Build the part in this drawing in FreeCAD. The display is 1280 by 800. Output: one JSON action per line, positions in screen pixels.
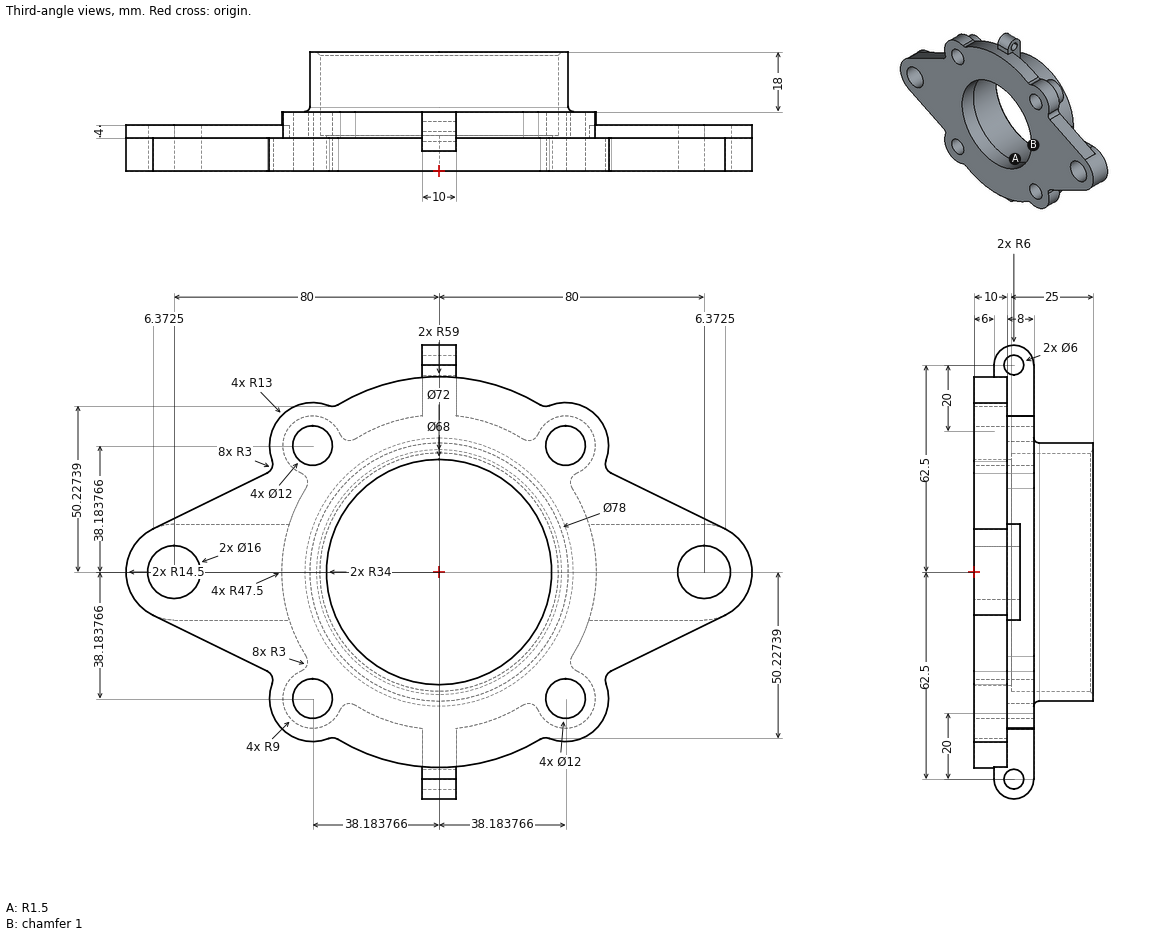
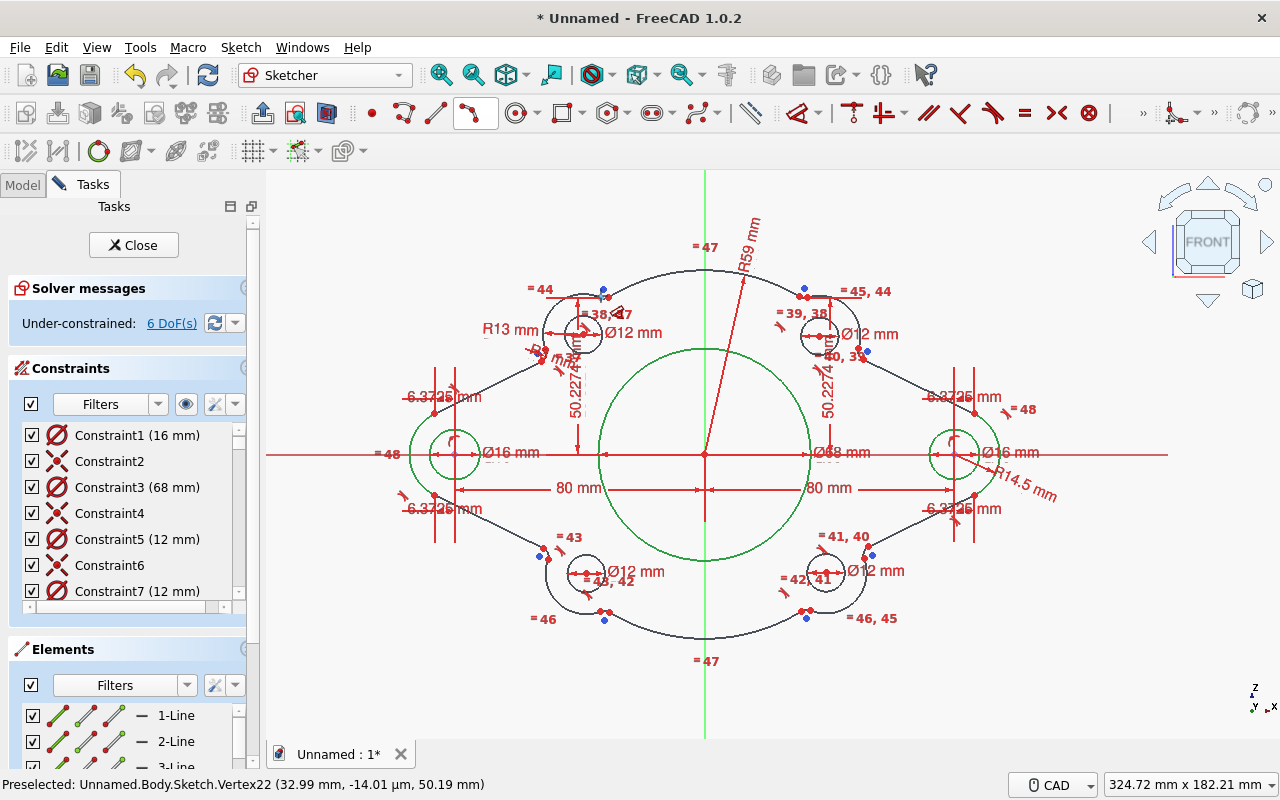
{"action": "scroll", "coordinate": [810, 610], "scroll_direction": "up", "scroll_amount": 2}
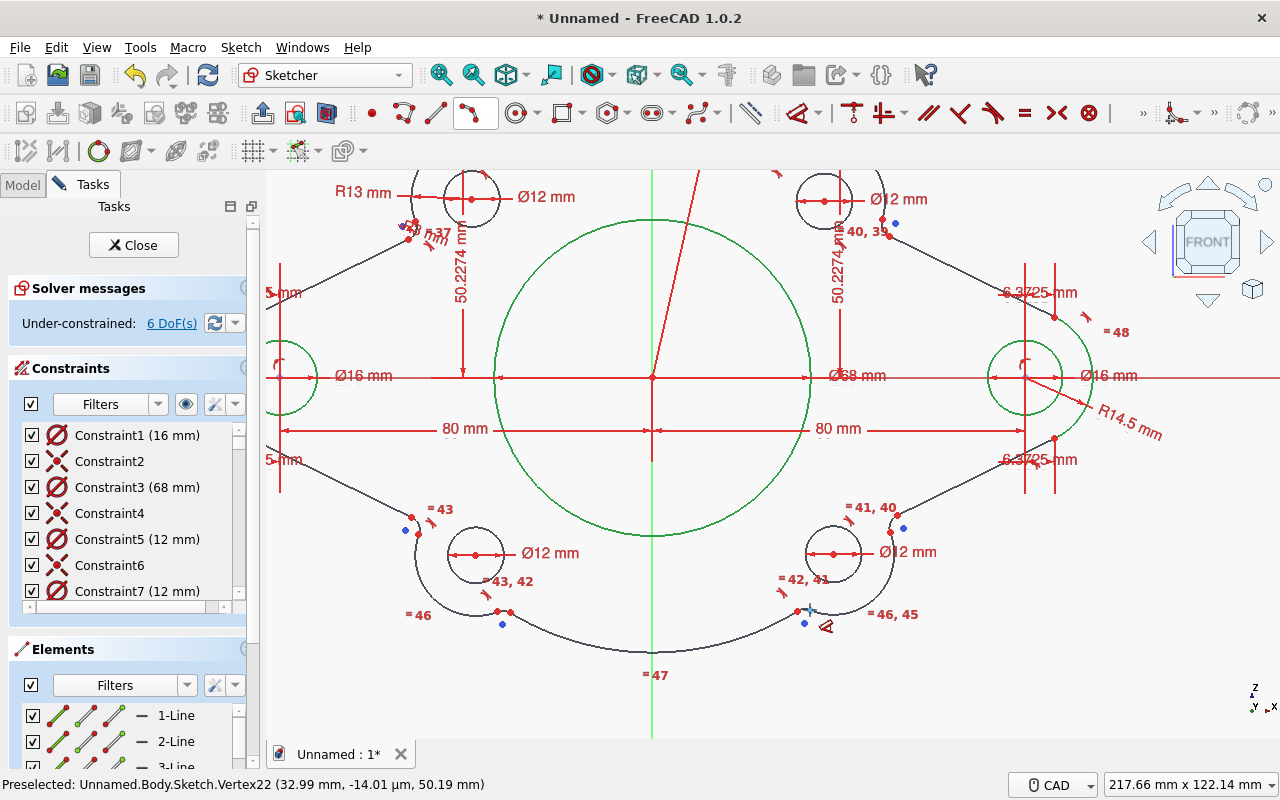
{"action": "left_click", "coordinate": [810, 610]}
{"action": "left_click", "coordinate": [844, 494]}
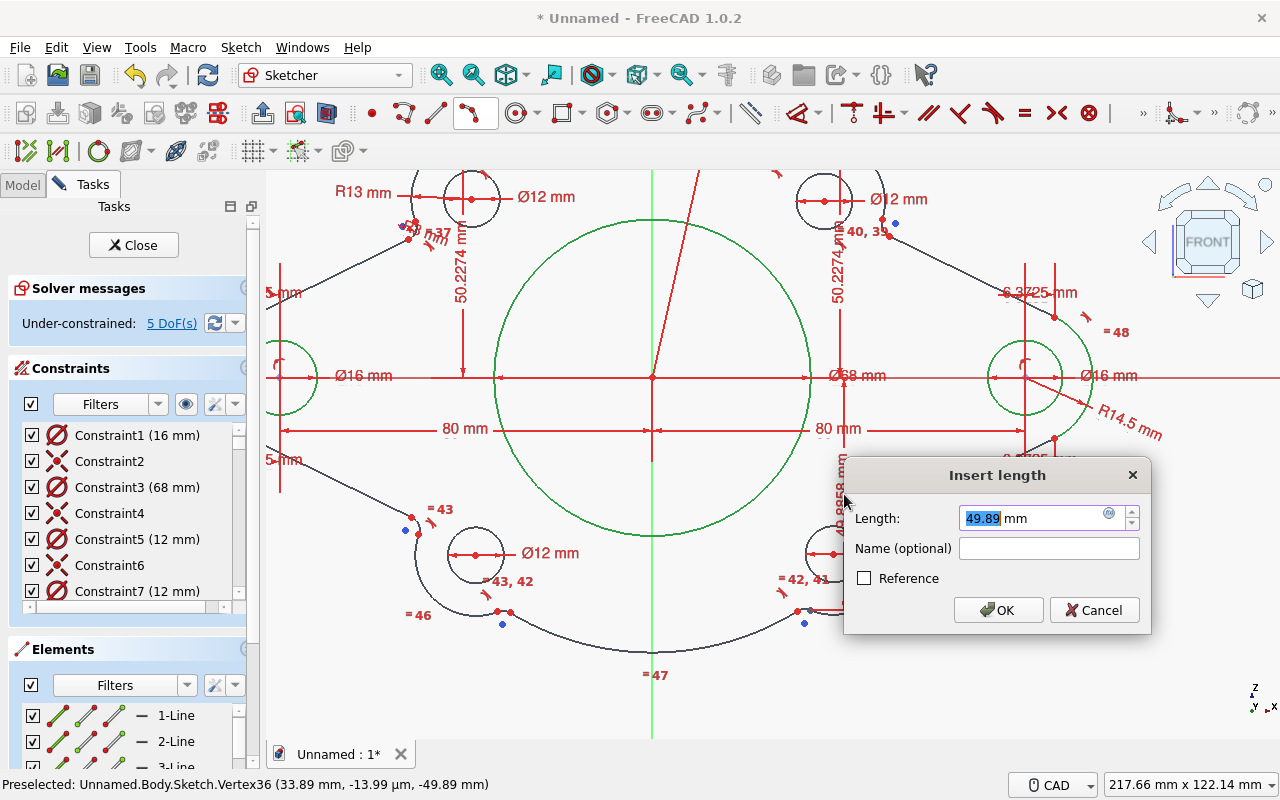
{"action": "type", "text": "50.22739"}
{"action": "key", "text": "Return"}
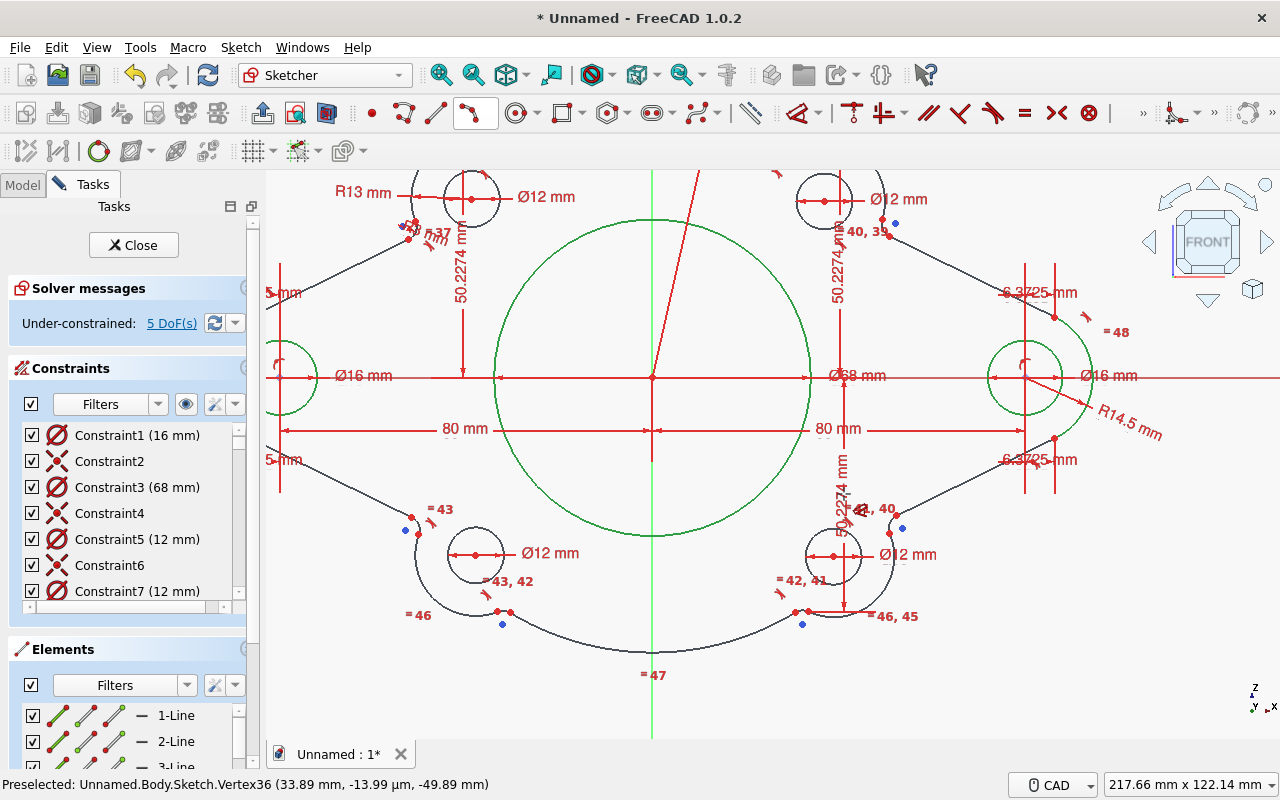
{"action": "left_click", "coordinate": [498, 612]}
{"action": "left_click", "coordinate": [464, 495]}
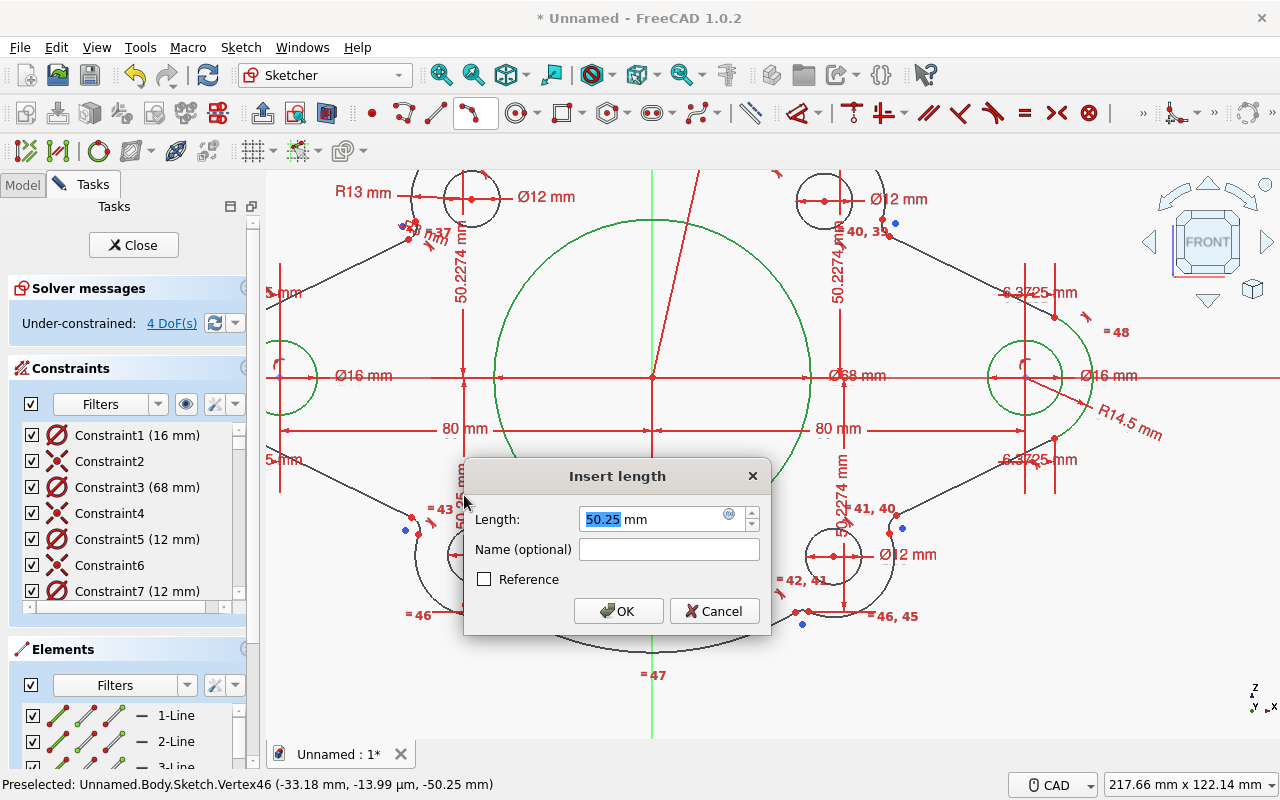
{"action": "type", "text": "50.22739"}
{"action": "key", "text": "Return"}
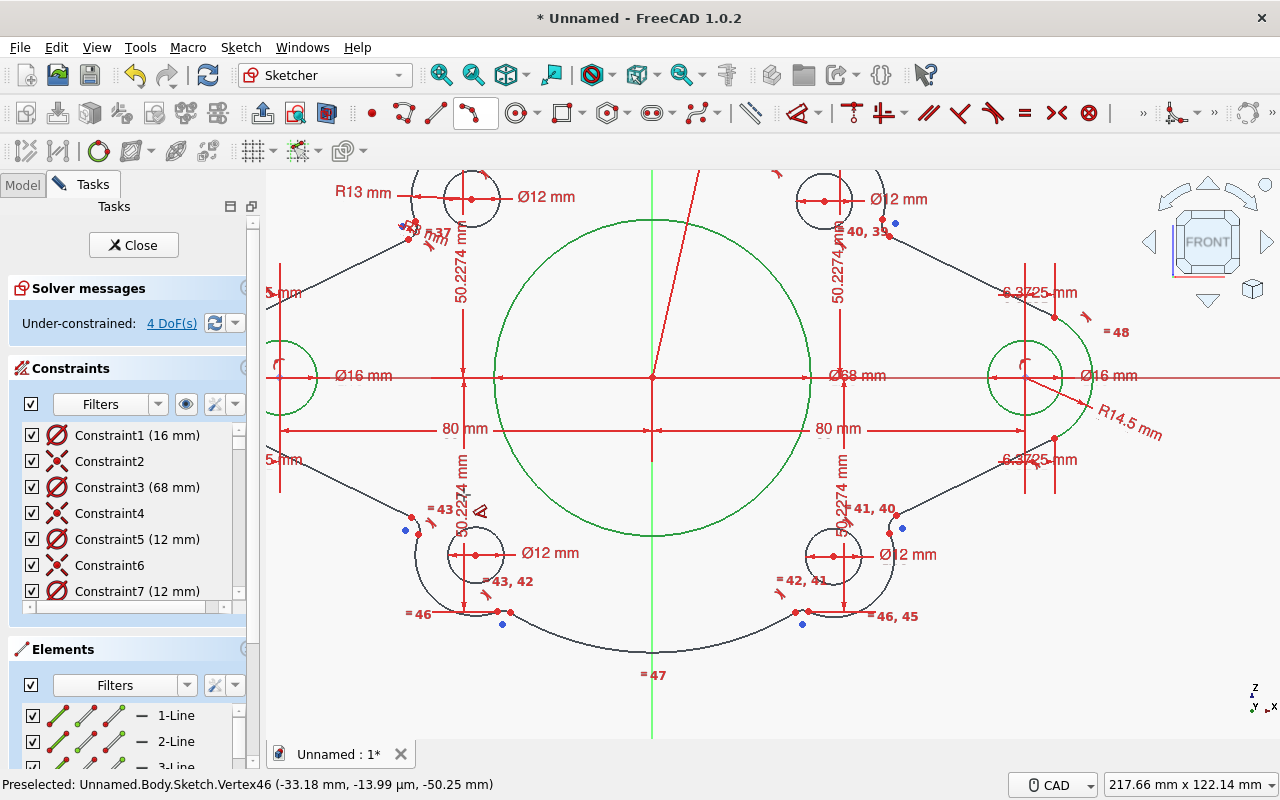
{"action": "left_click", "coordinate": [834, 557]}
{"action": "left_click", "coordinate": [743, 591]}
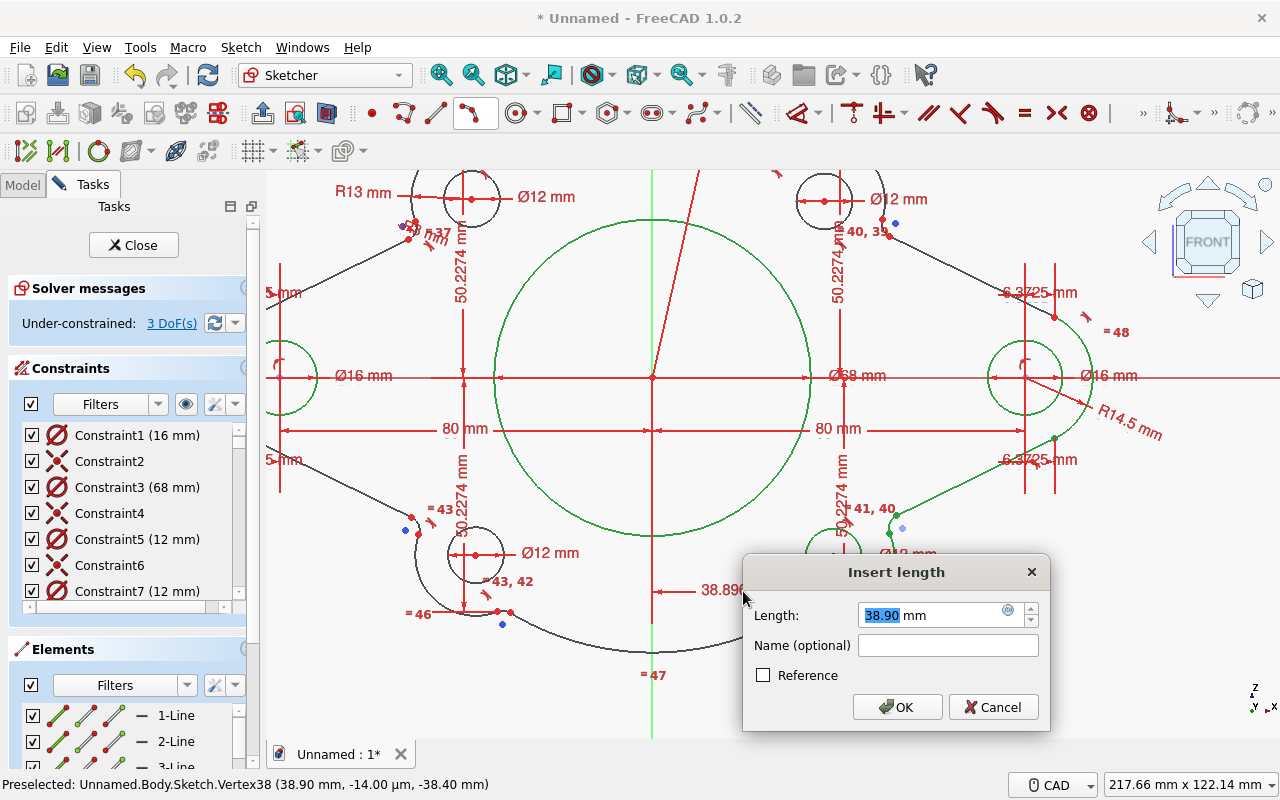
{"action": "type", "text": "38.183766"}
{"action": "key", "text": "Return"}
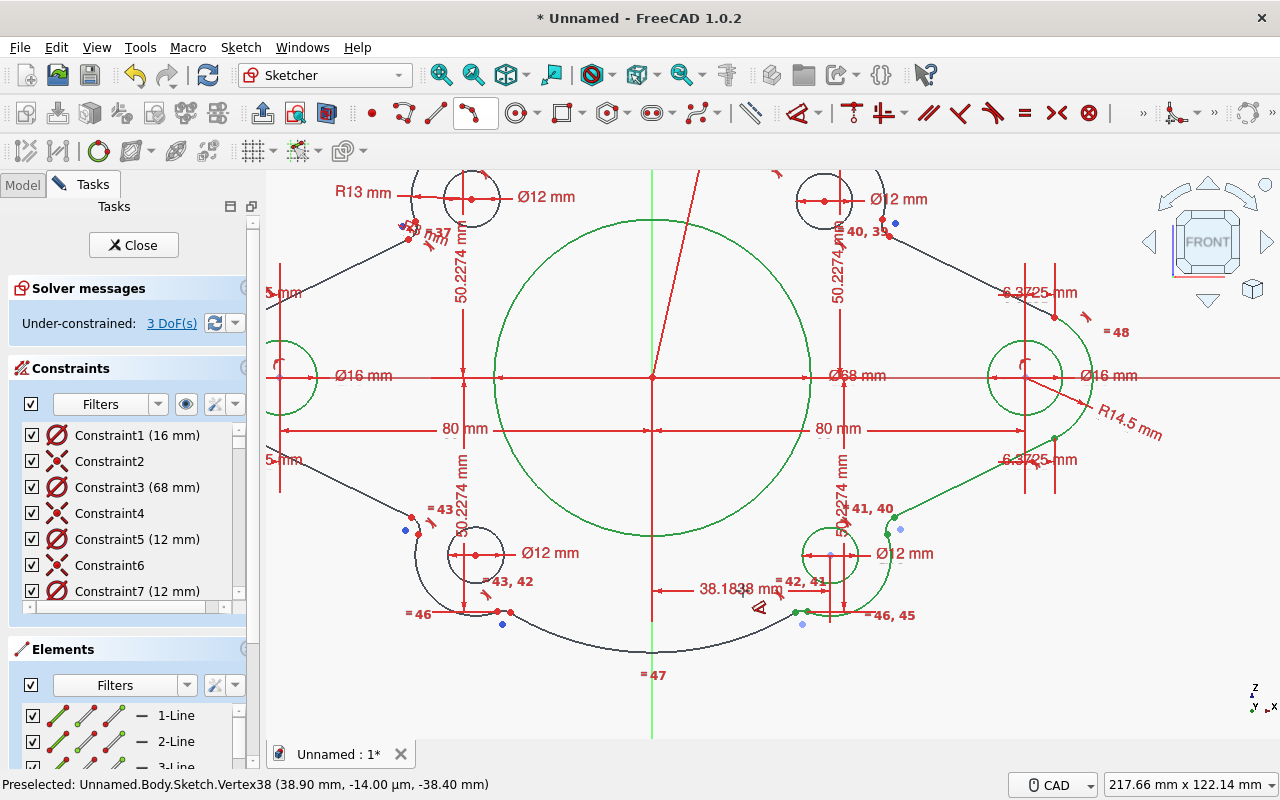
{"action": "left_click", "coordinate": [476, 555]}
{"action": "left_click", "coordinate": [564, 589]}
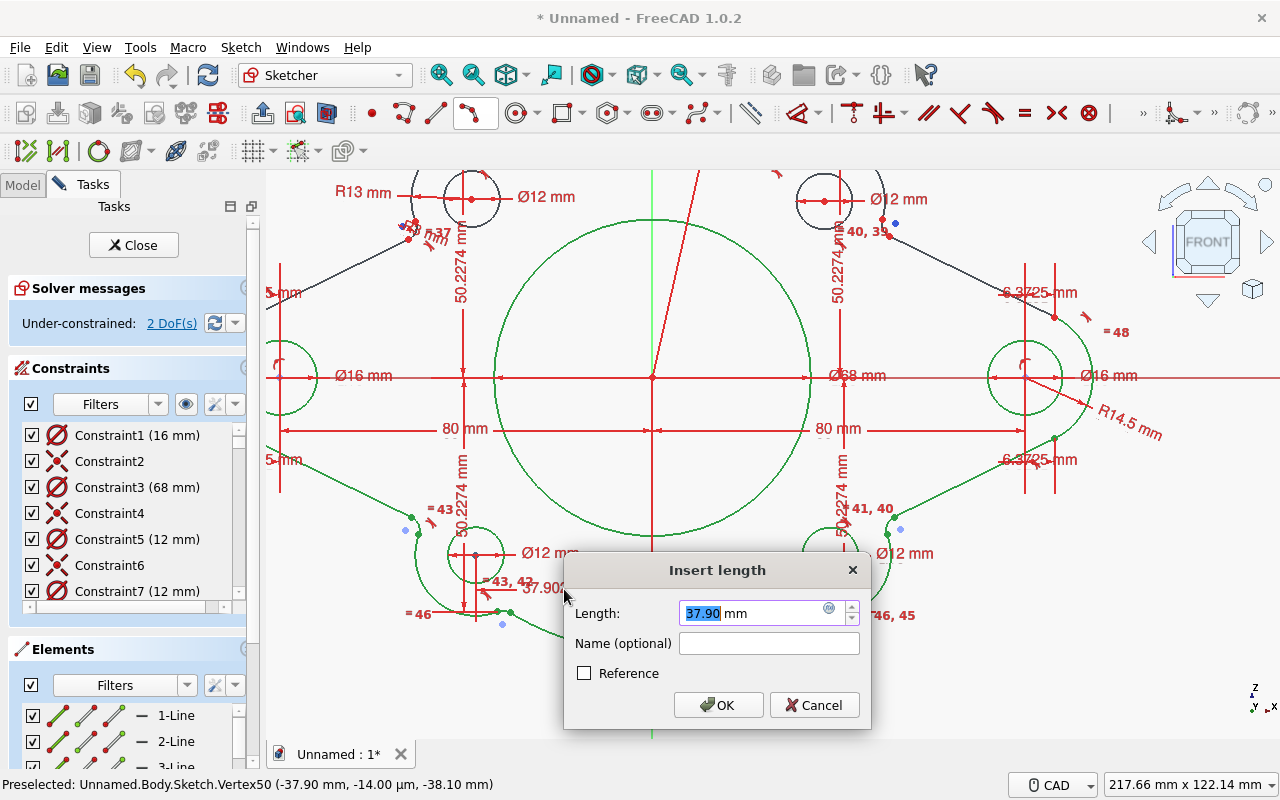
{"action": "type", "text": "38.183766"}
{"action": "key", "text": "Return"}